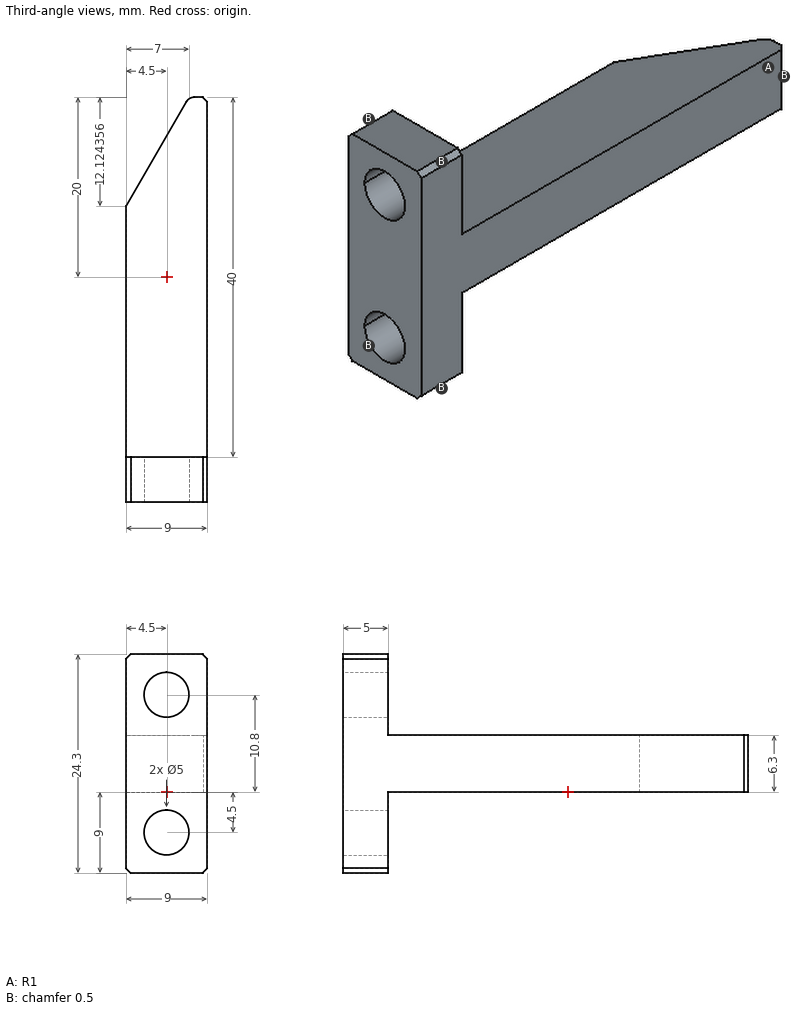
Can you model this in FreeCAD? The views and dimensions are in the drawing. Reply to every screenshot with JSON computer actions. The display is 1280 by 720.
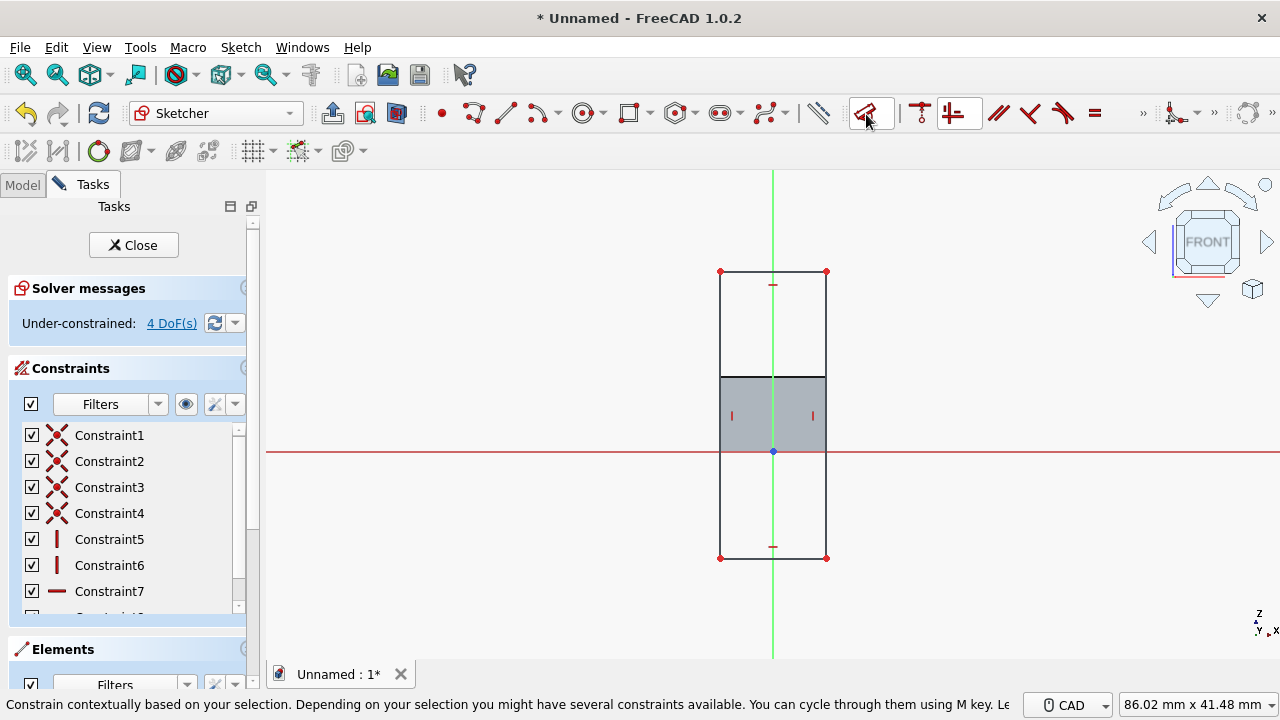
{"action": "left_click", "coordinate": [752, 559]}
{"action": "left_click", "coordinate": [749, 593]}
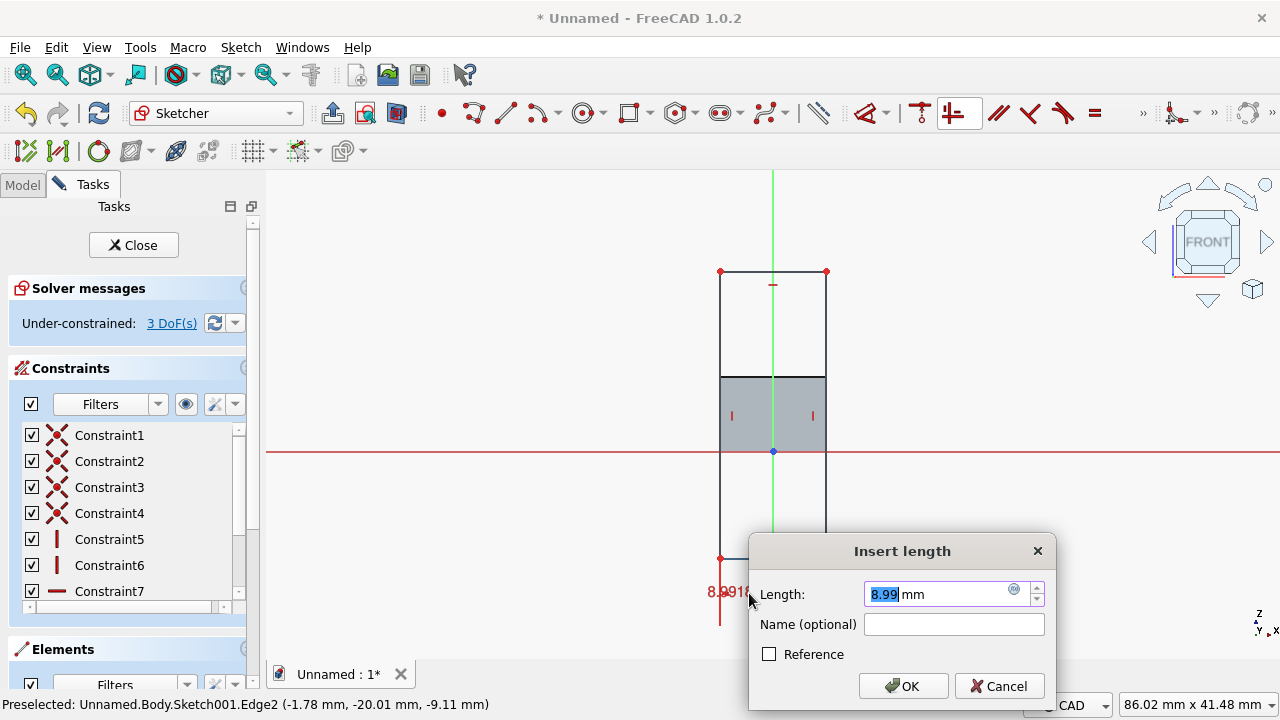
{"action": "type", "text": "9"}
{"action": "key", "text": "Return"}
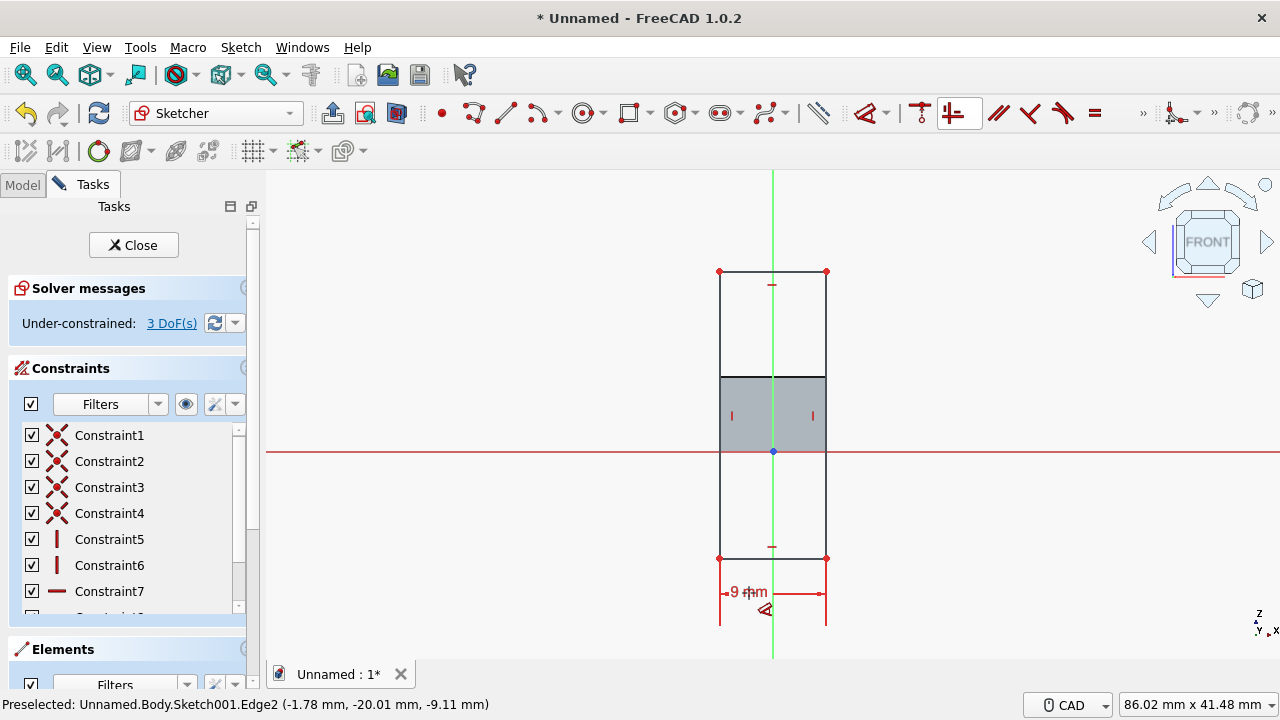
{"action": "left_click", "coordinate": [720, 559]}
{"action": "left_click", "coordinate": [686, 505]}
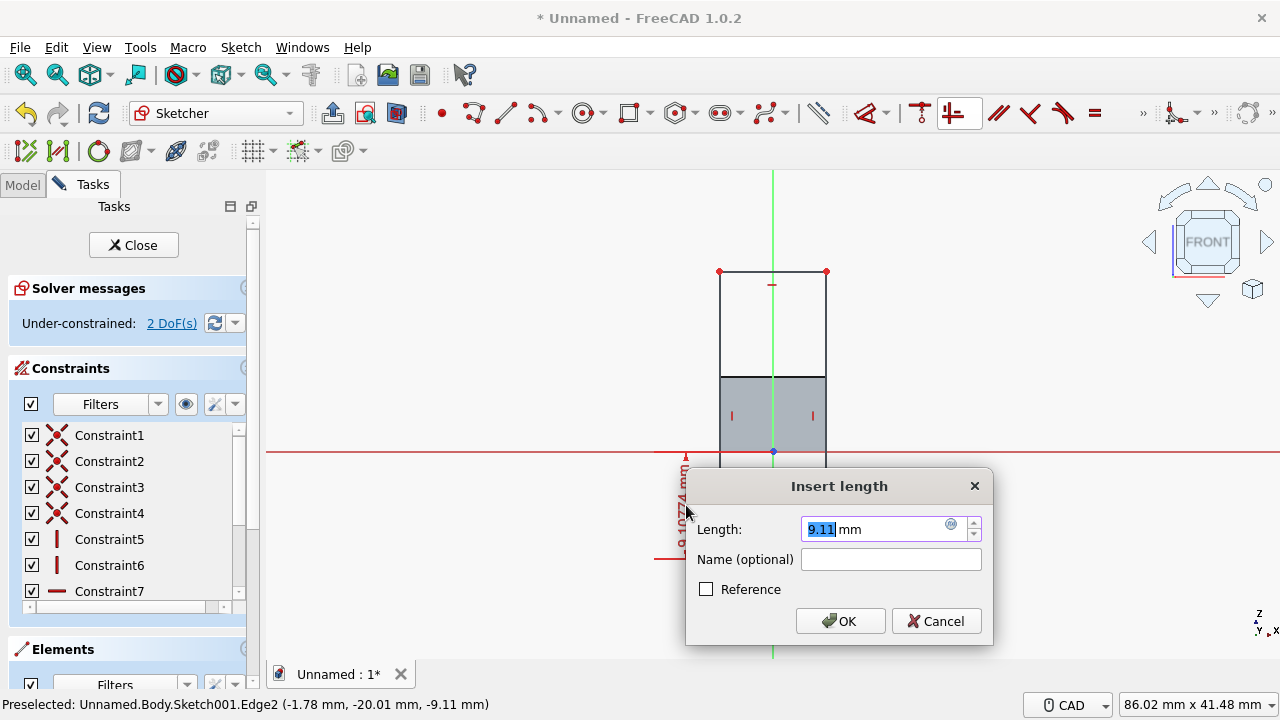
{"action": "type", "text": "9"}
{"action": "key", "text": "Return"}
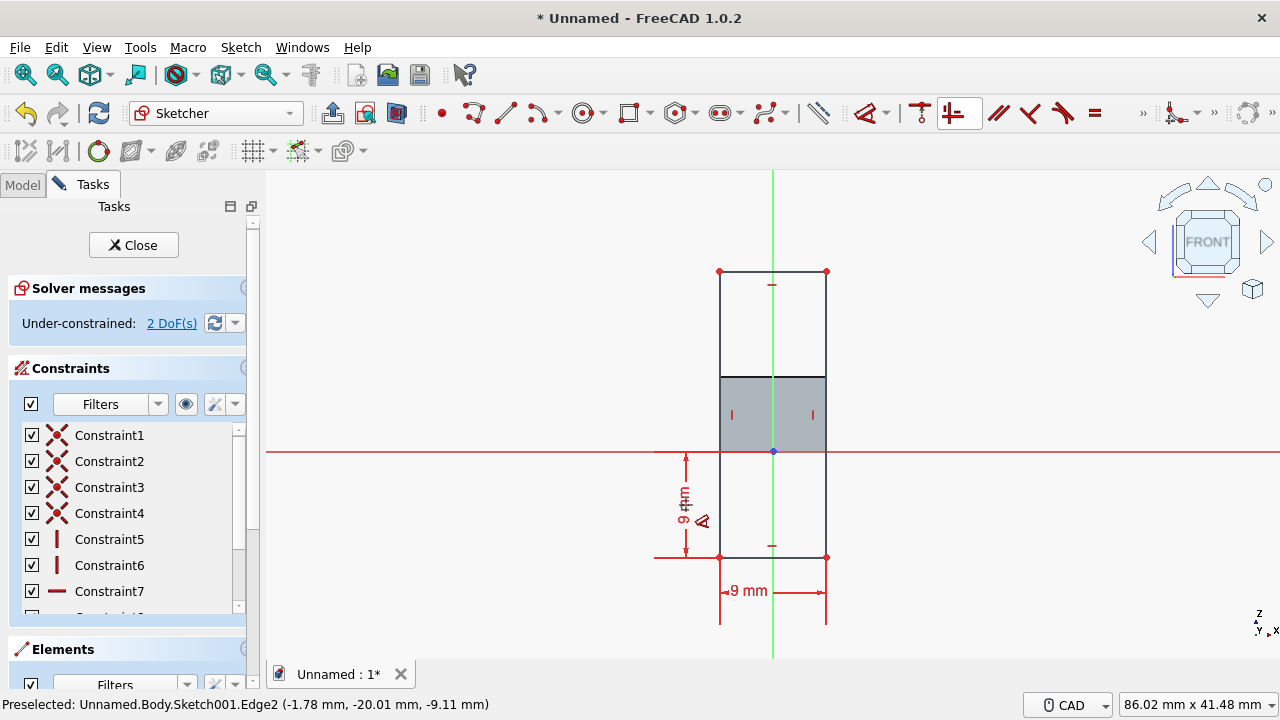
{"action": "left_click", "coordinate": [720, 358]}
{"action": "left_click", "coordinate": [686, 415]}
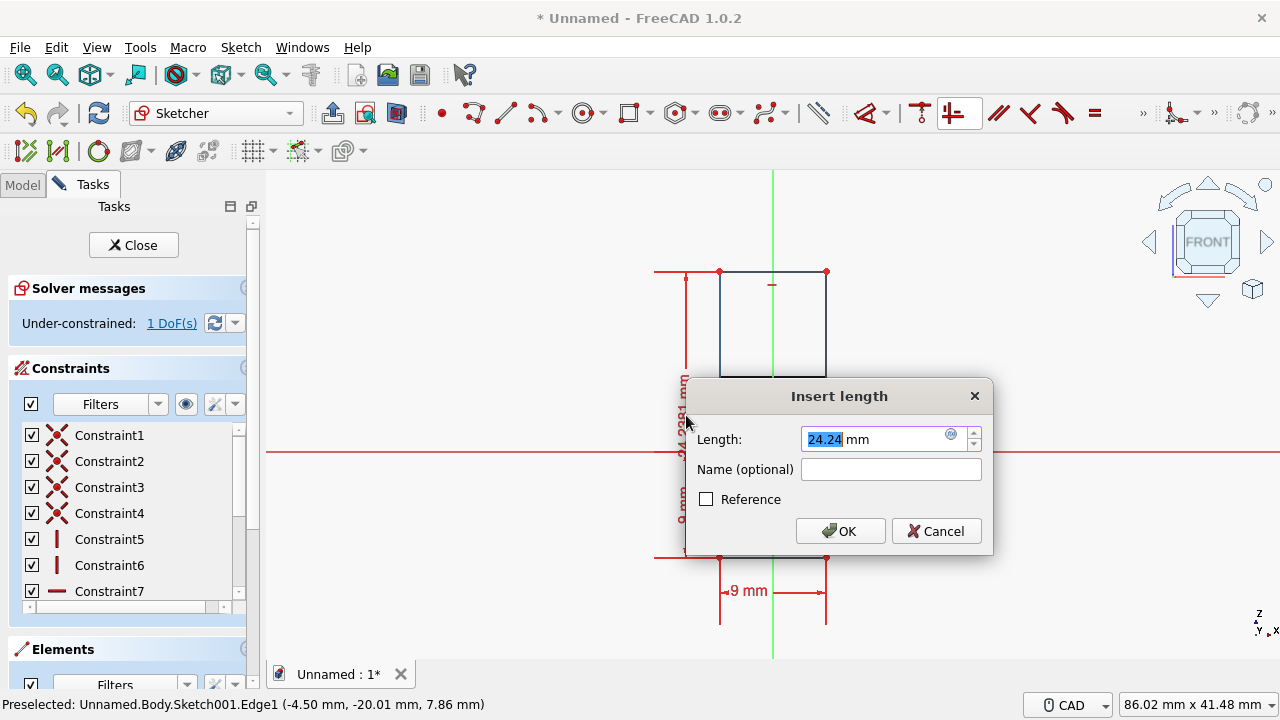
{"action": "type", "text": "24.3"}
{"action": "key", "text": "Return"}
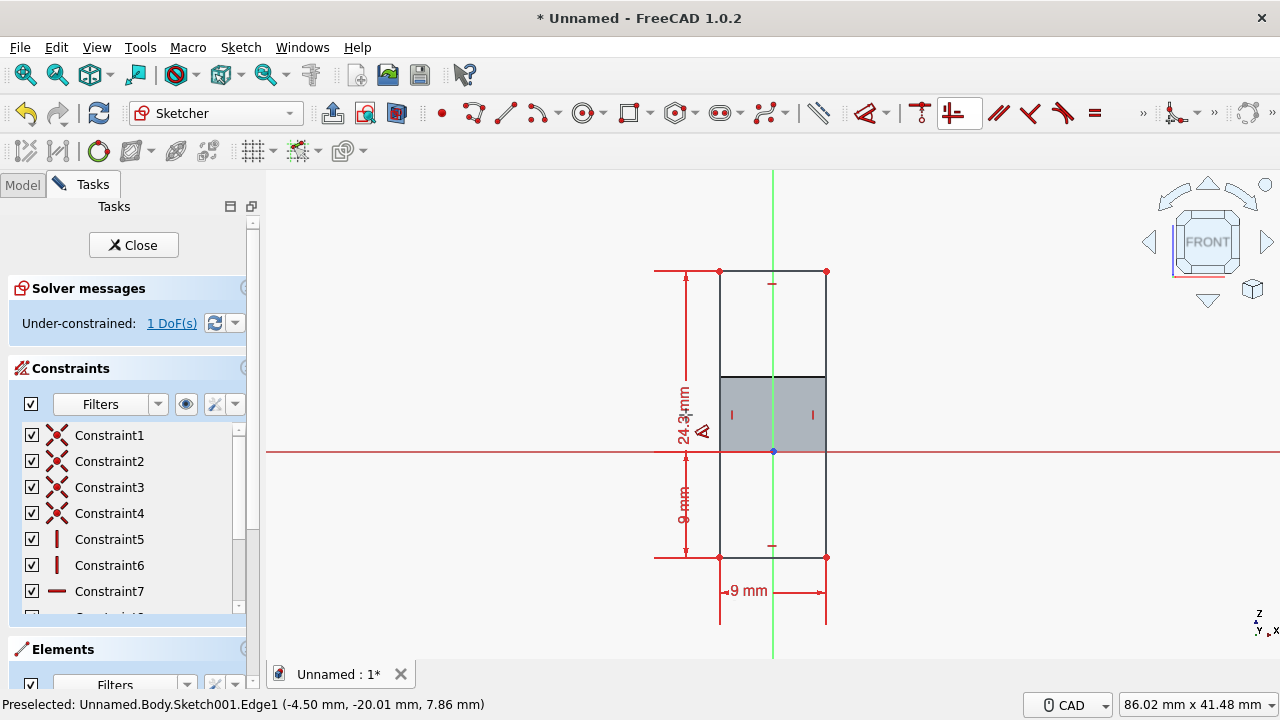
{"action": "left_click", "coordinate": [720, 271]}
{"action": "left_click", "coordinate": [746, 237]}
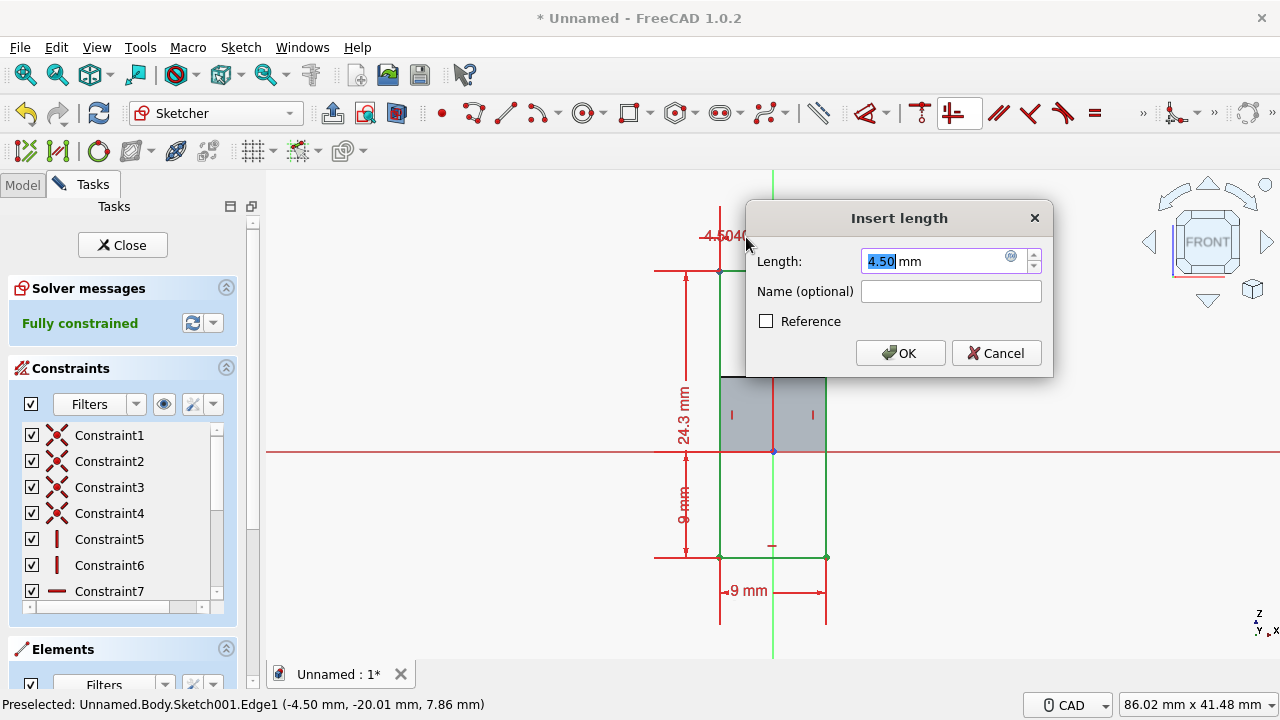
{"action": "type", "text": "4.5"}
{"action": "key", "text": "Return"}
{"action": "key", "text": "Escape"}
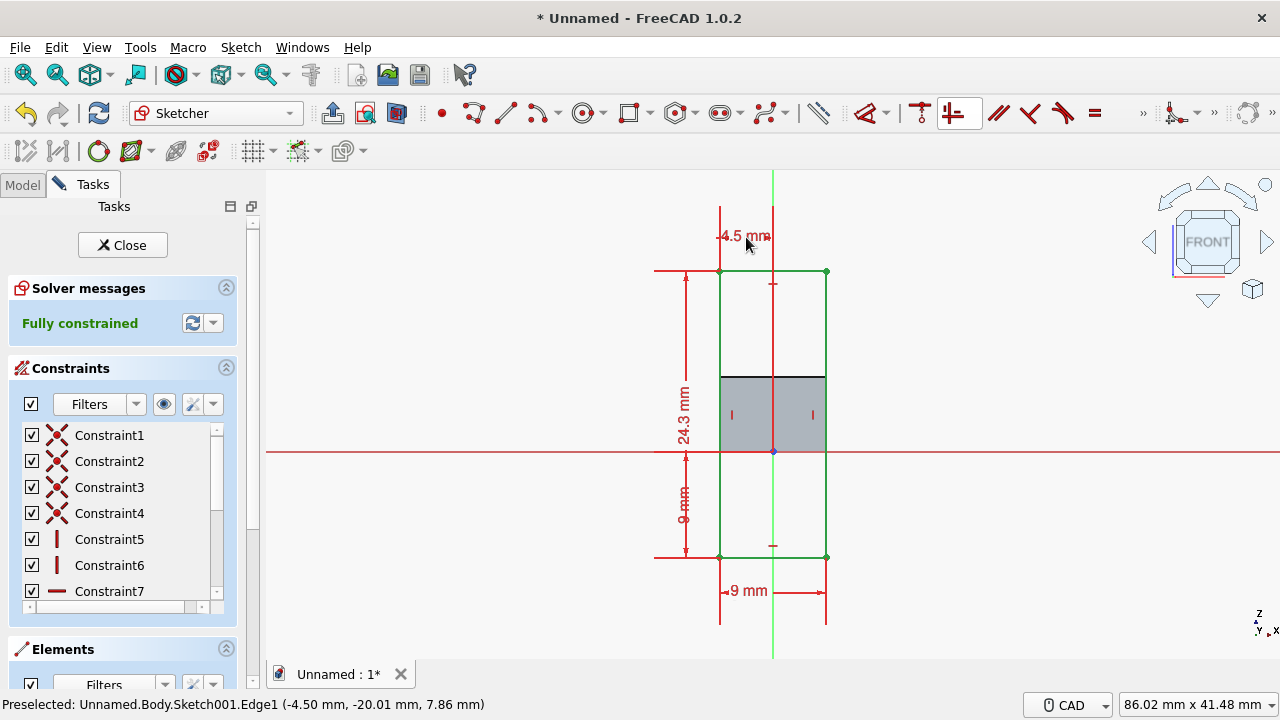
{"action": "left_click", "coordinate": [123, 245]}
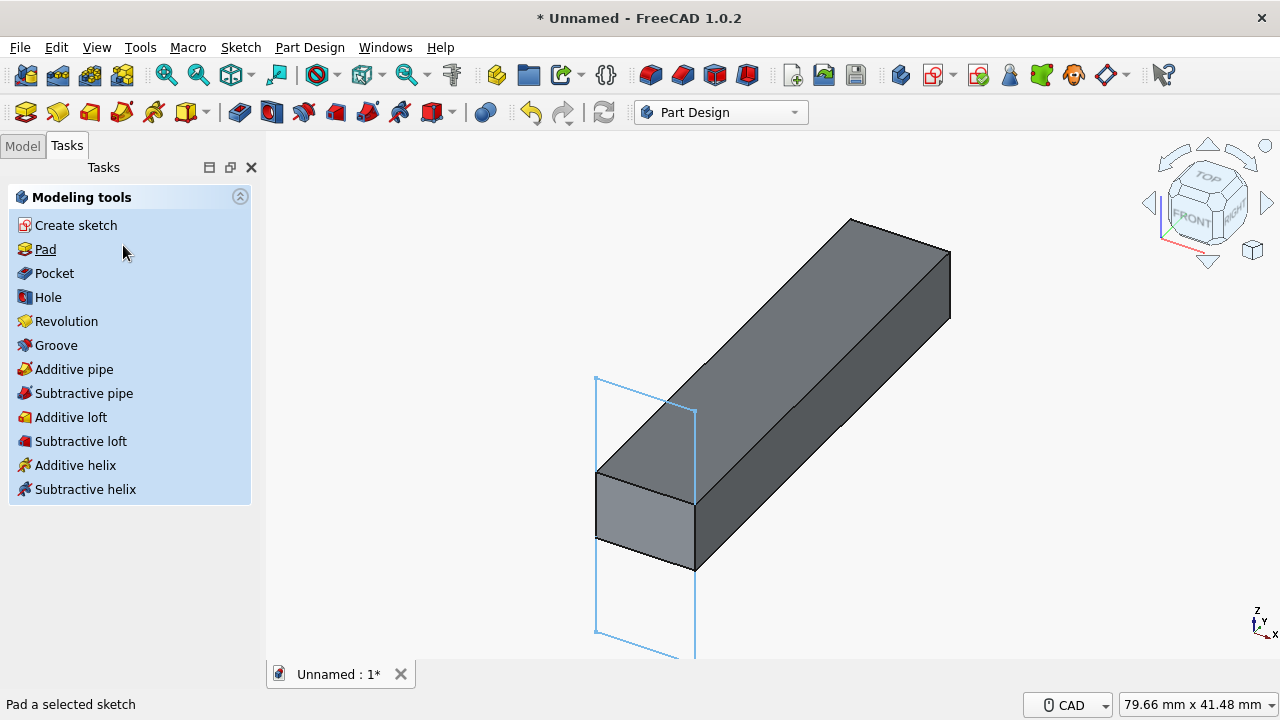
{"action": "left_click", "coordinate": [26, 112]}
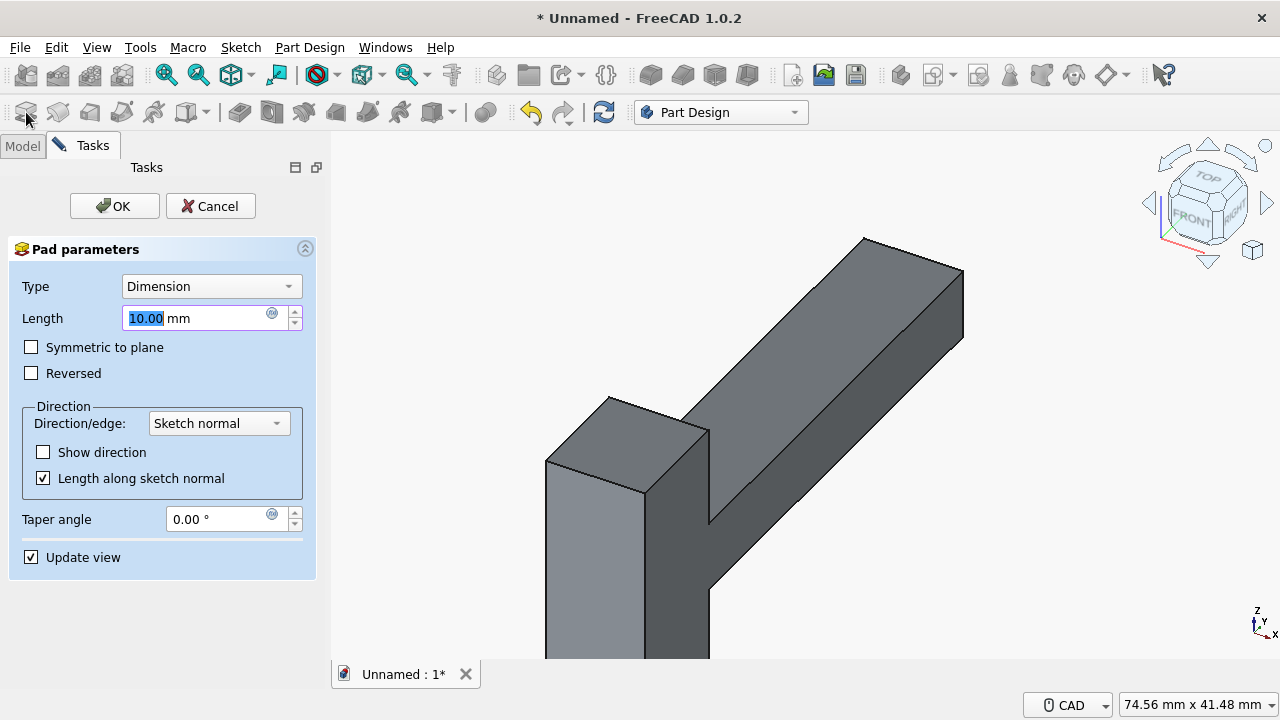
{"action": "type", "text": "5"}
{"action": "key", "text": "Tab"}